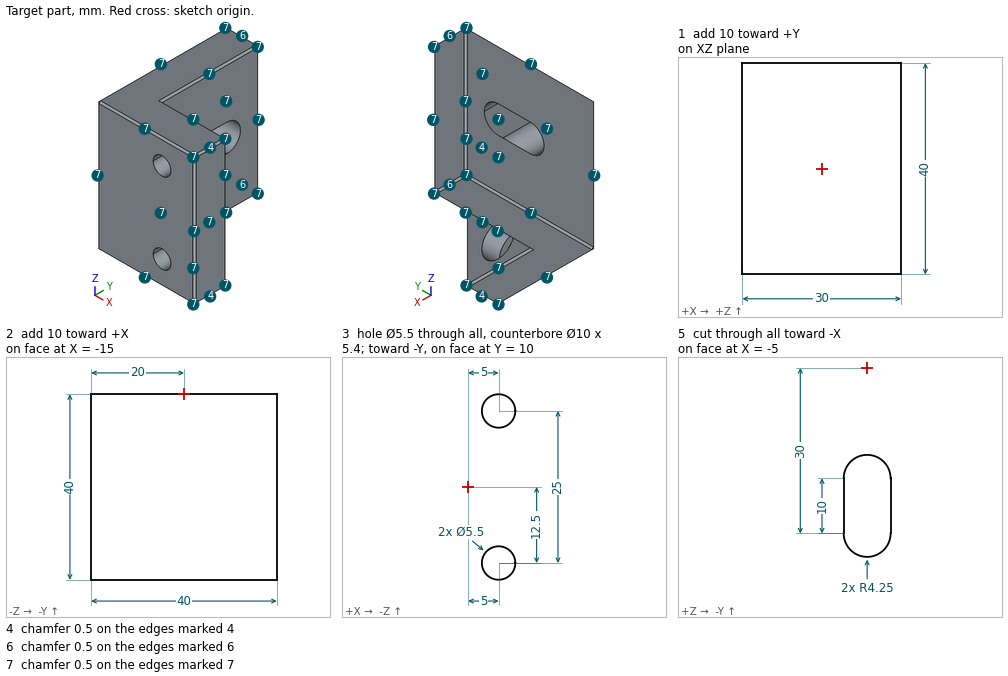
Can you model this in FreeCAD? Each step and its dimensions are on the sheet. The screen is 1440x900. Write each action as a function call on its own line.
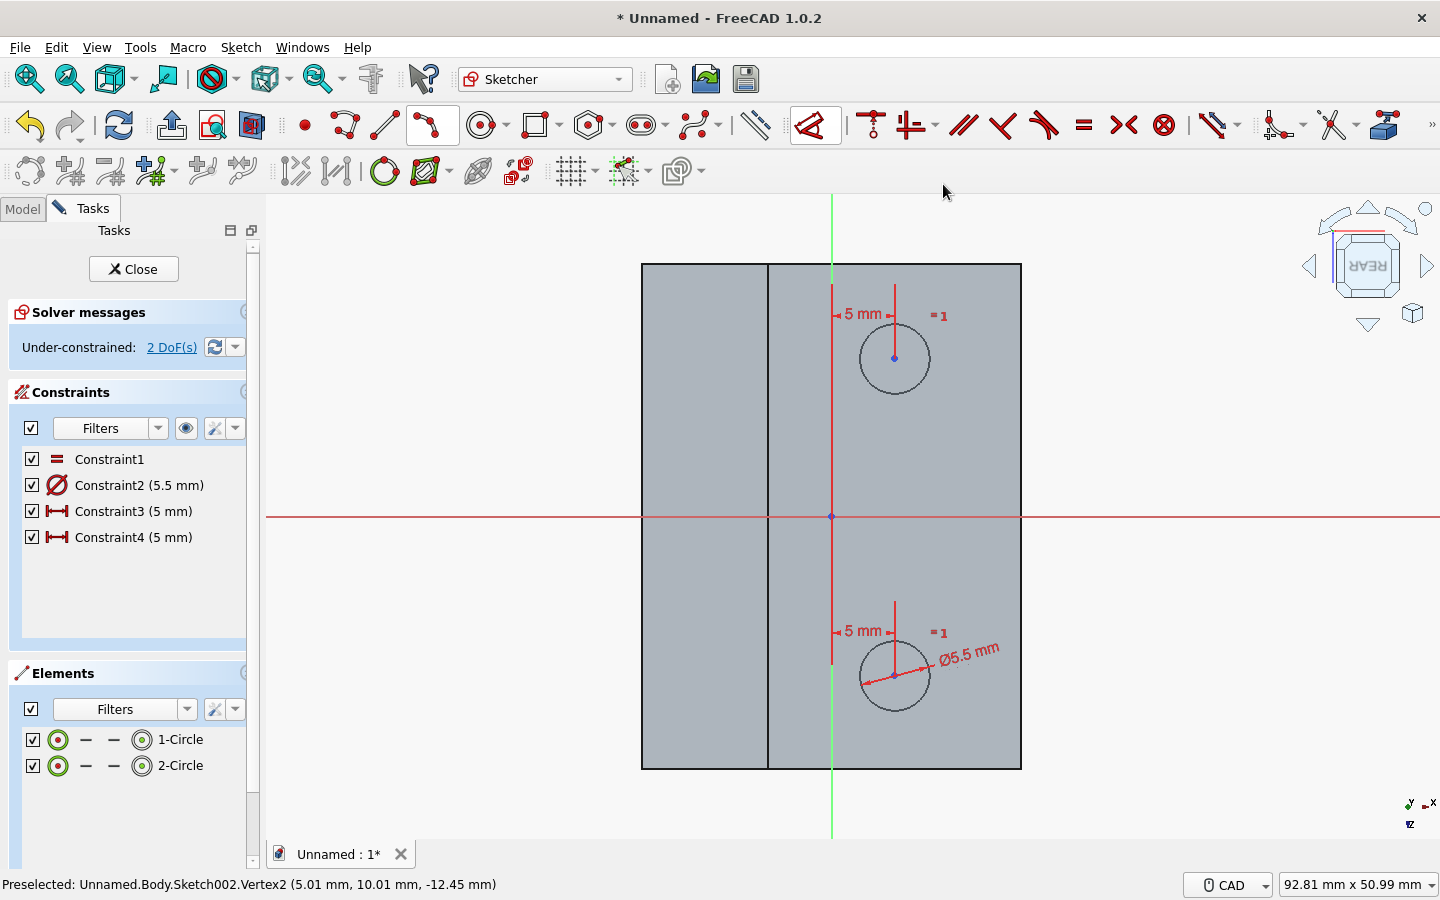
click(895, 676)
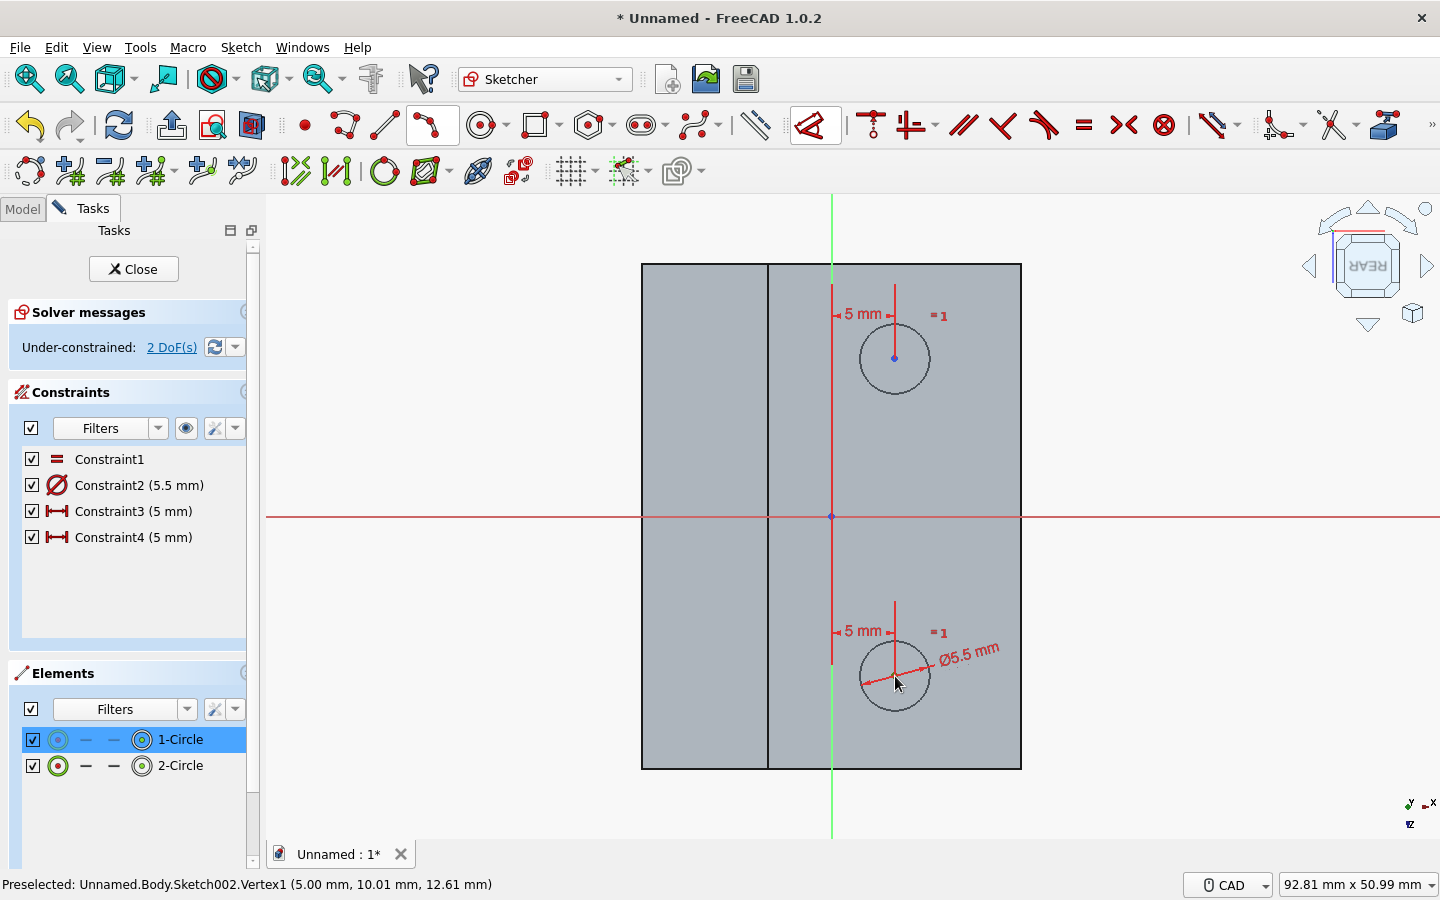
click(895, 359)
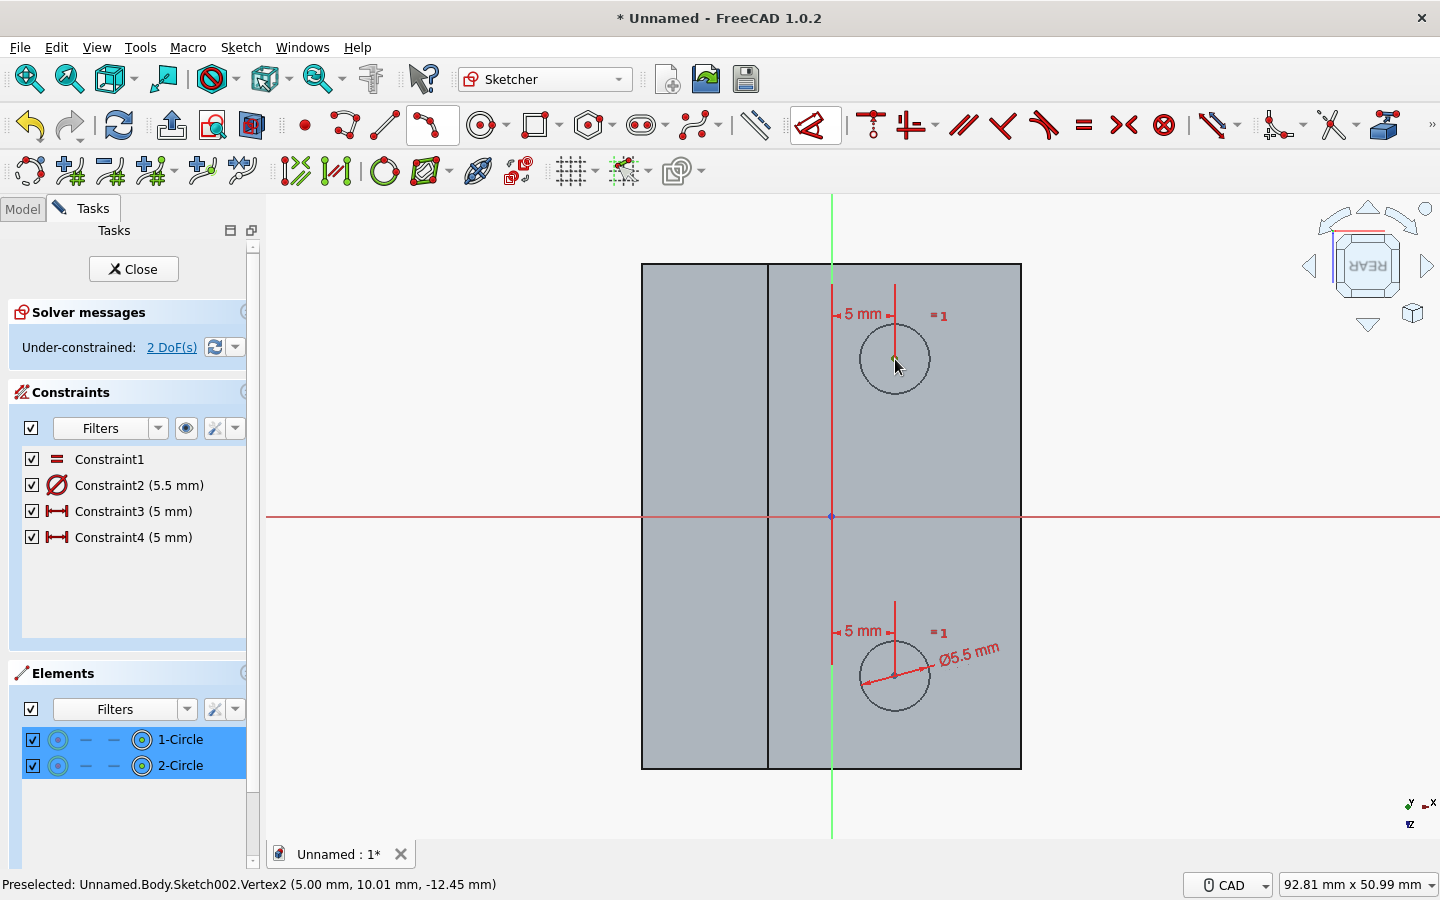
key(i)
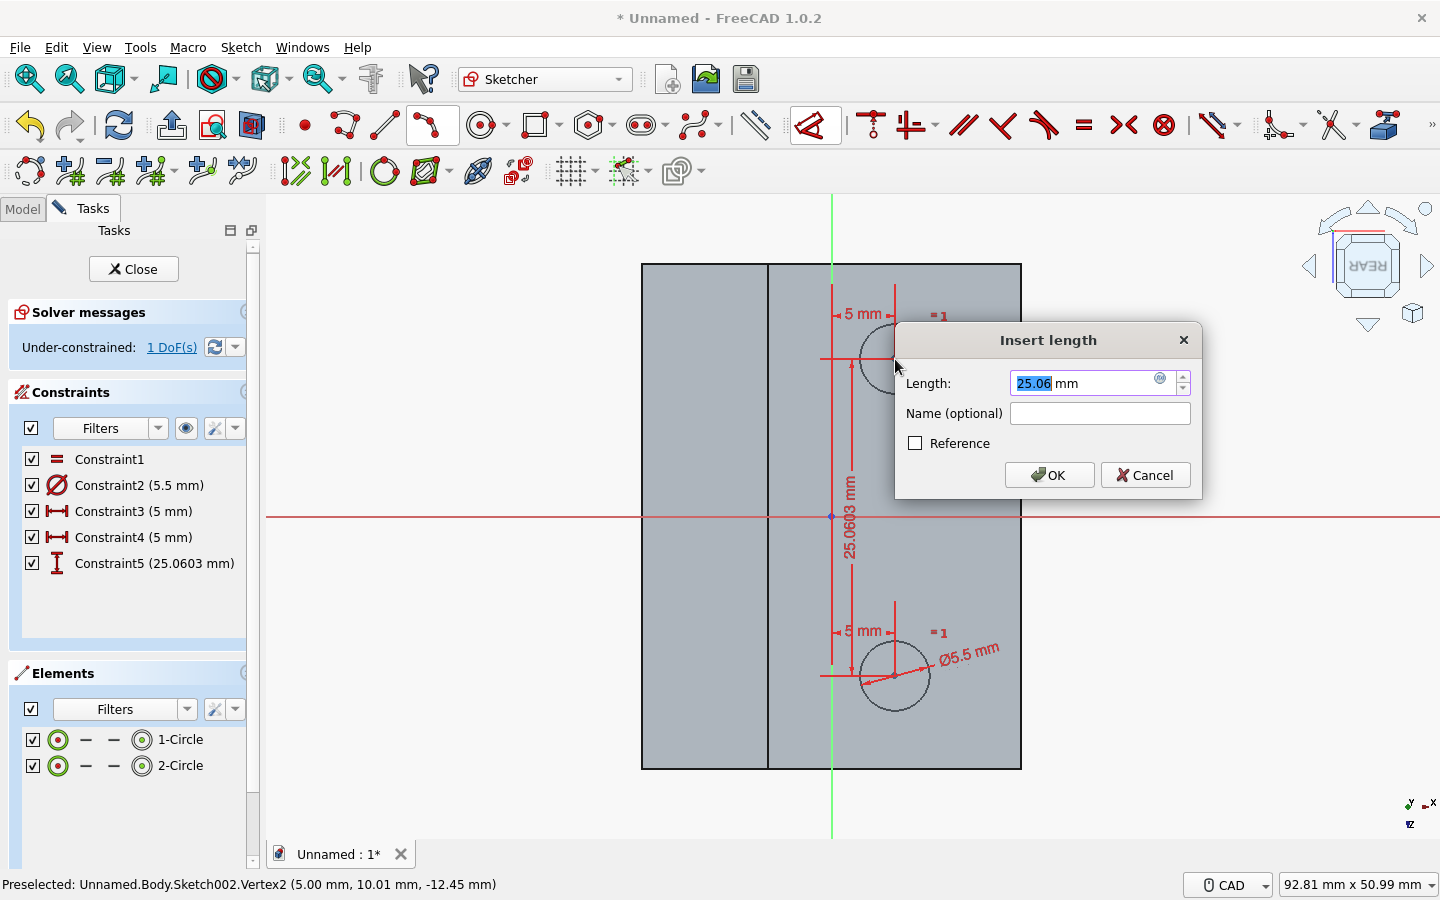
text(25)
key(Return)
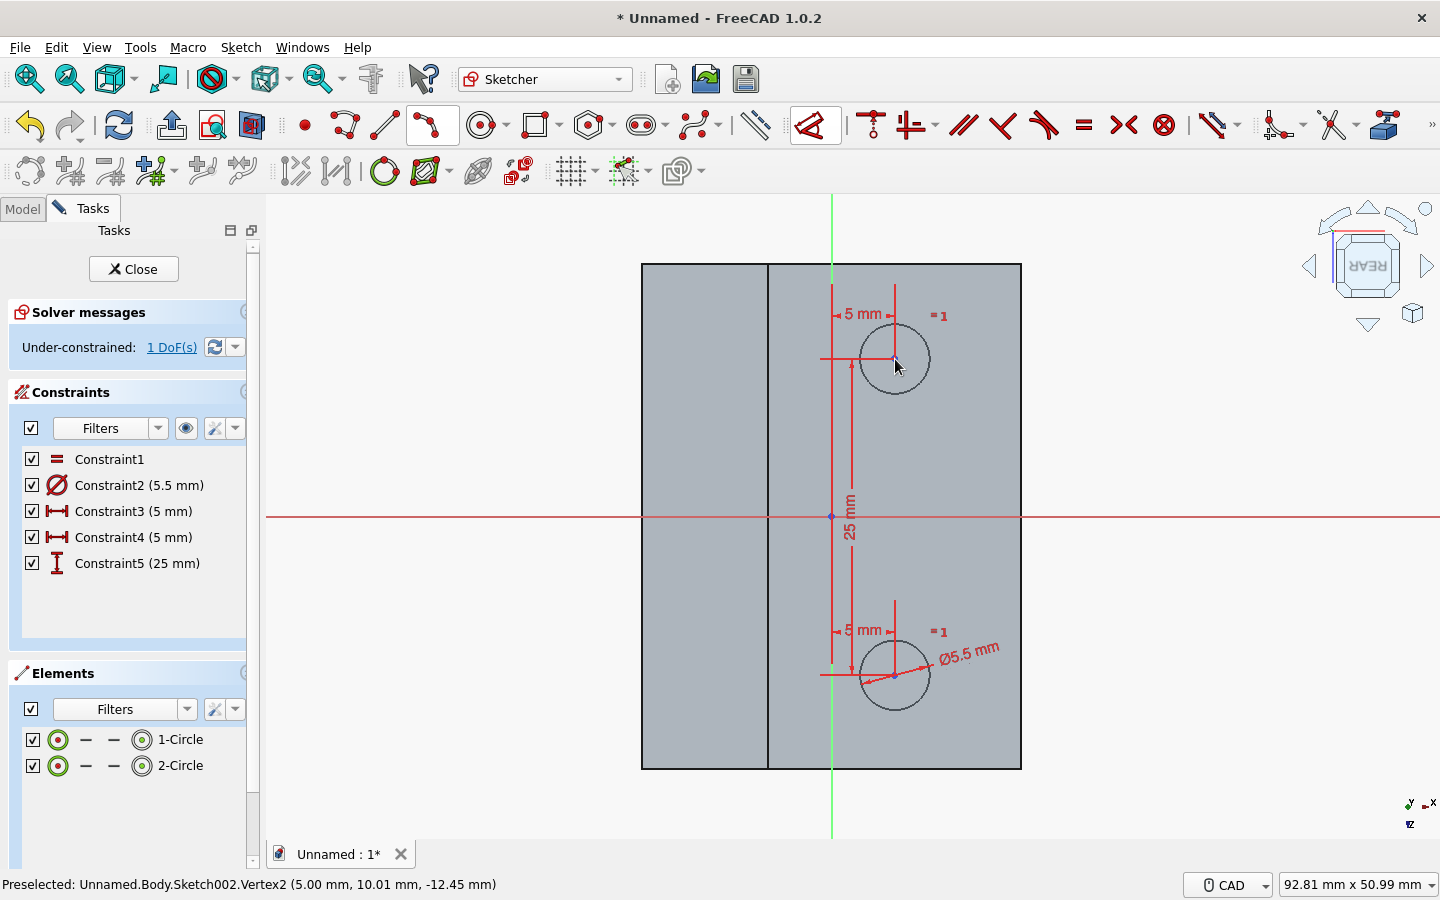
click(895, 675)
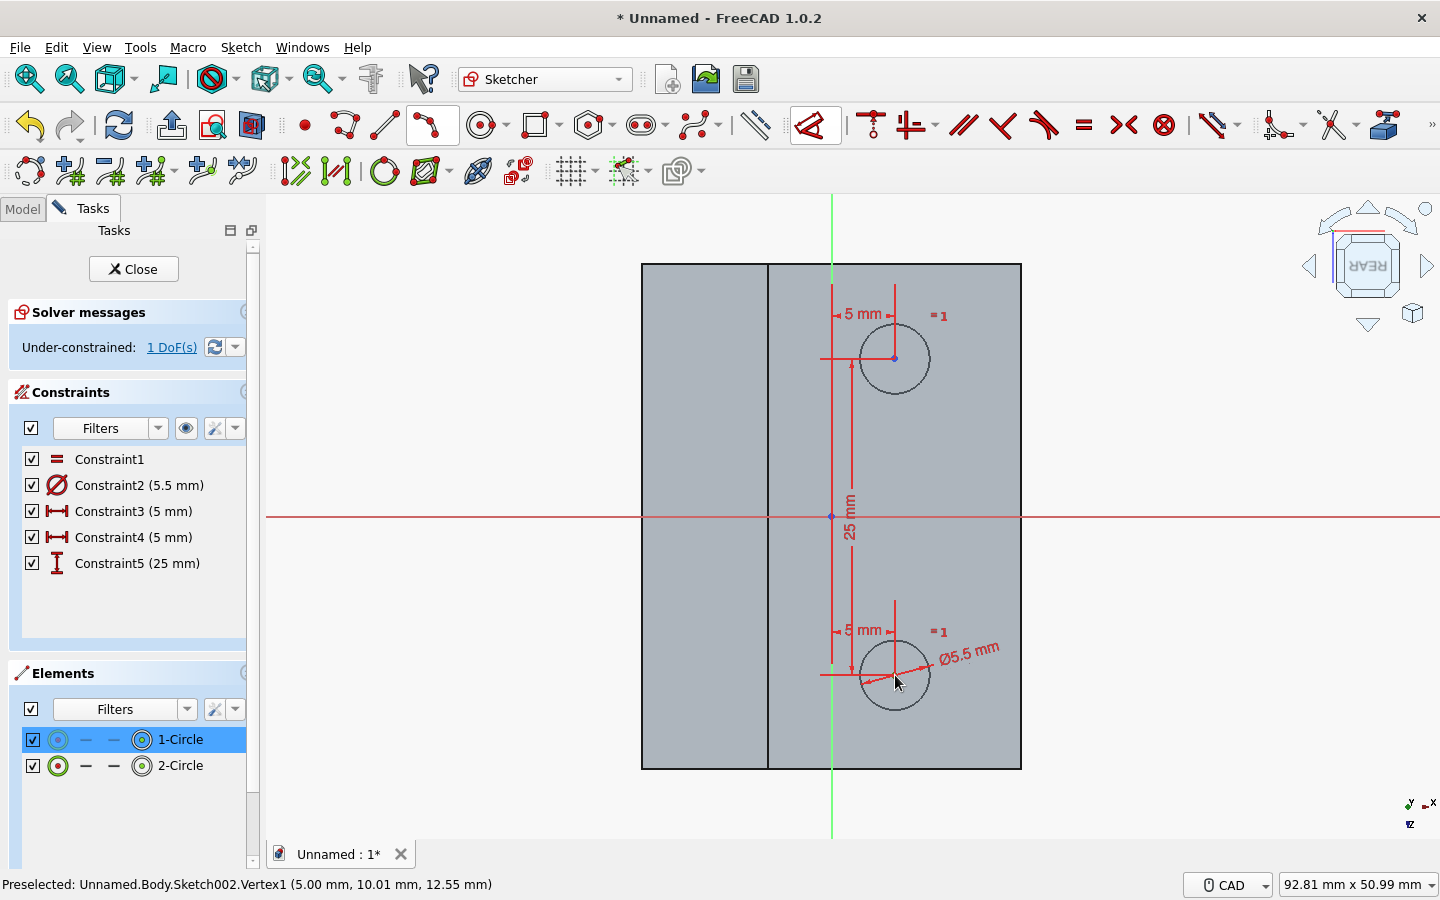
key(i)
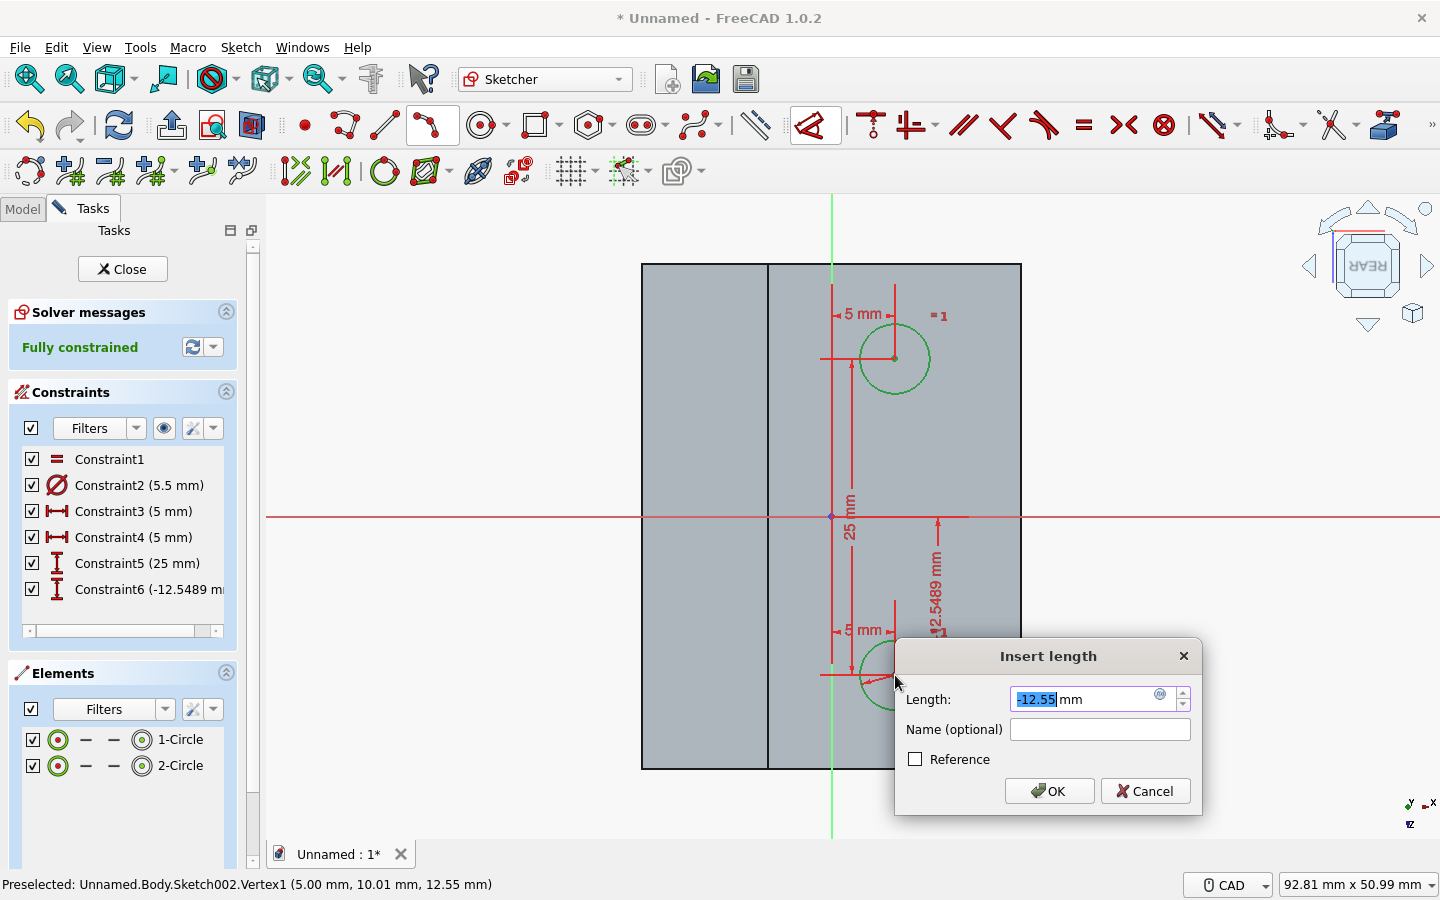
text(-12.5)
key(Return)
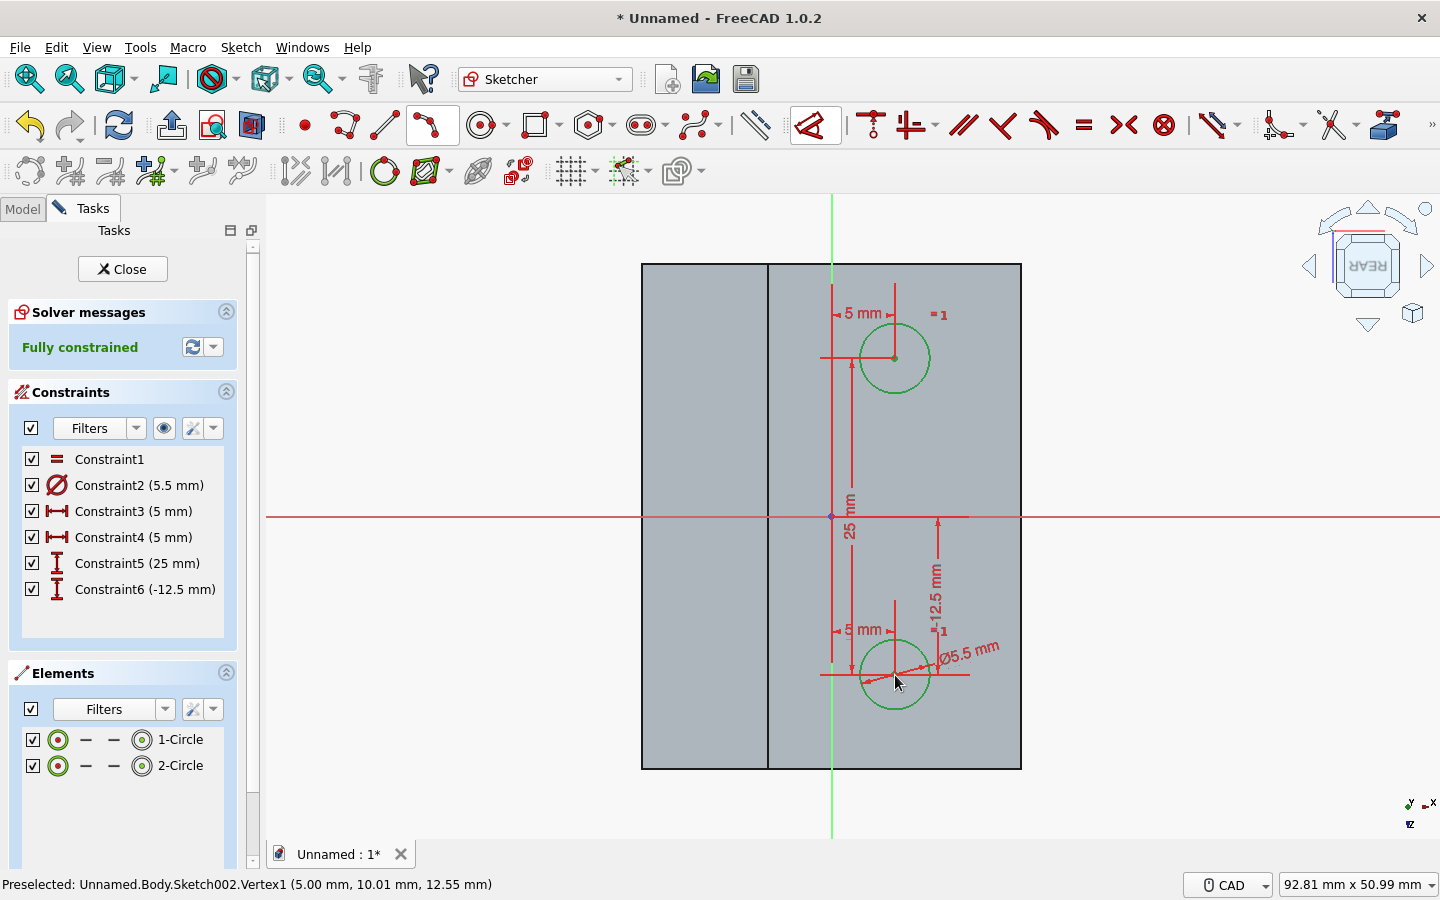
click(123, 269)